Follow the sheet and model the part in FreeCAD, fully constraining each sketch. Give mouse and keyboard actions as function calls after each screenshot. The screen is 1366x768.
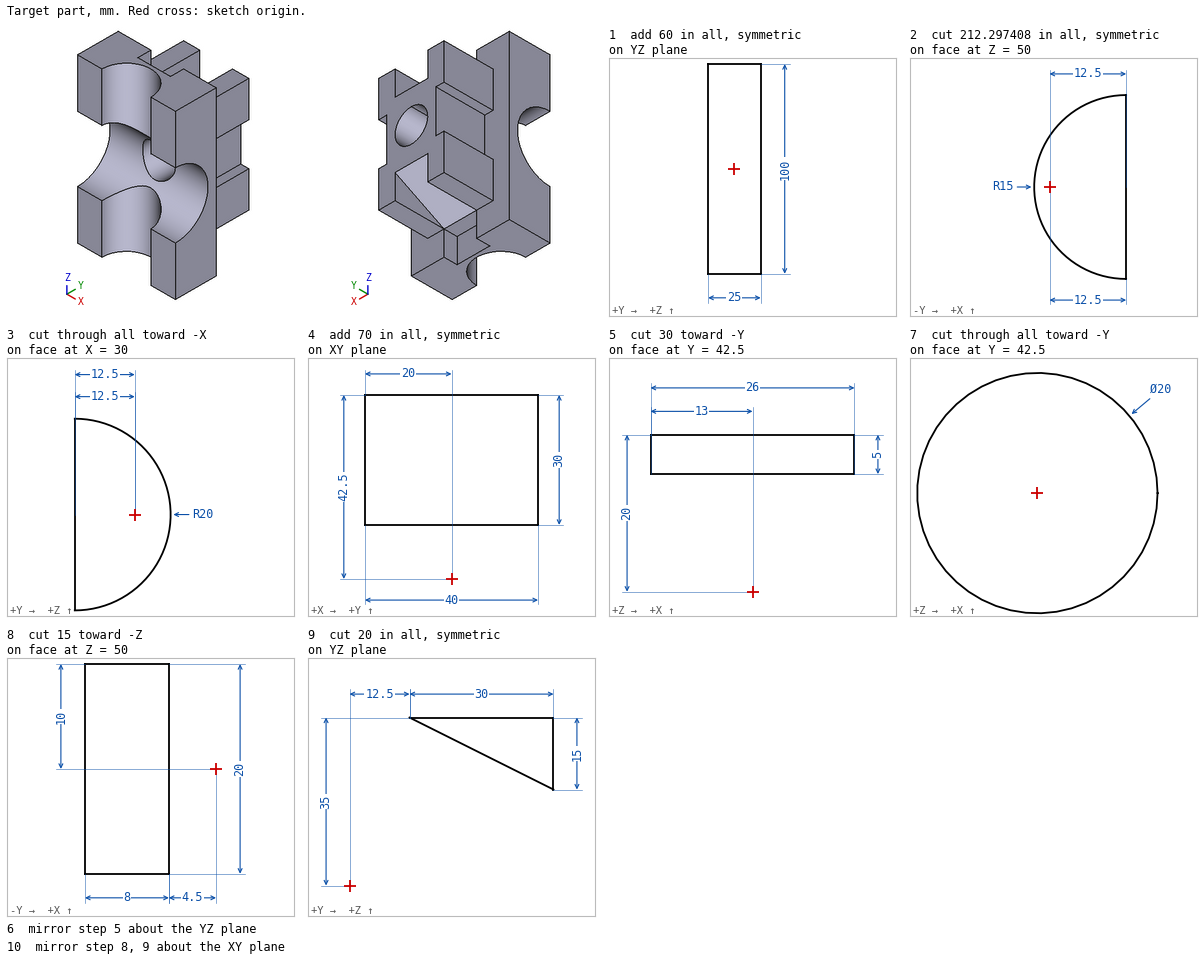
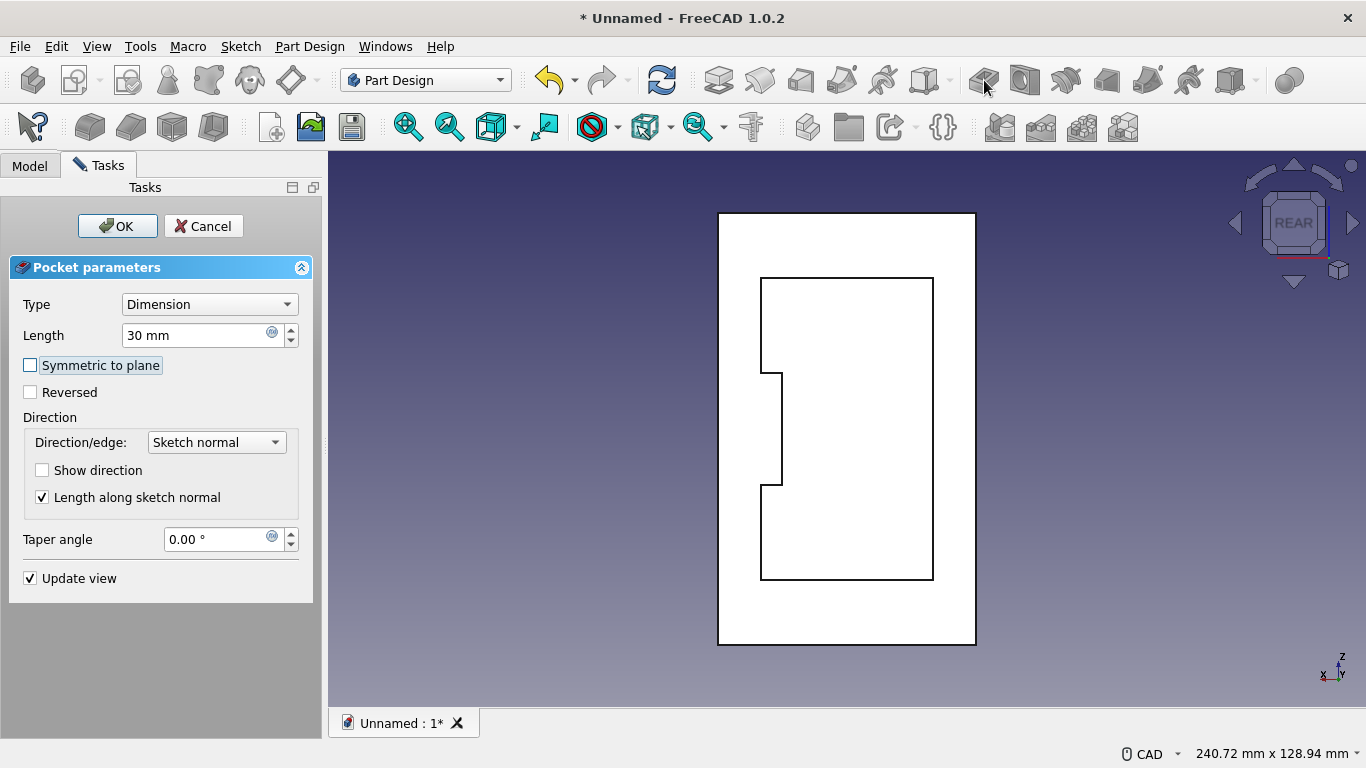
click(118, 226)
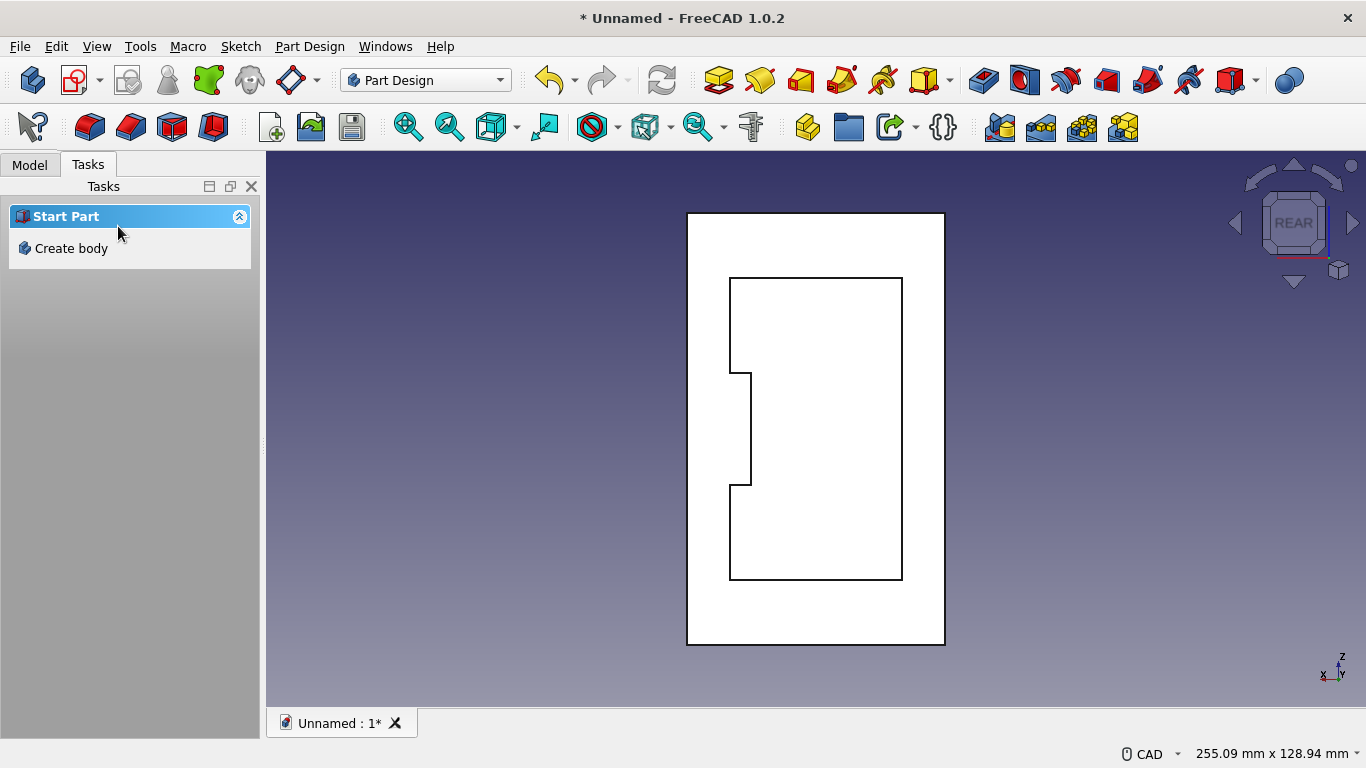
click(30, 164)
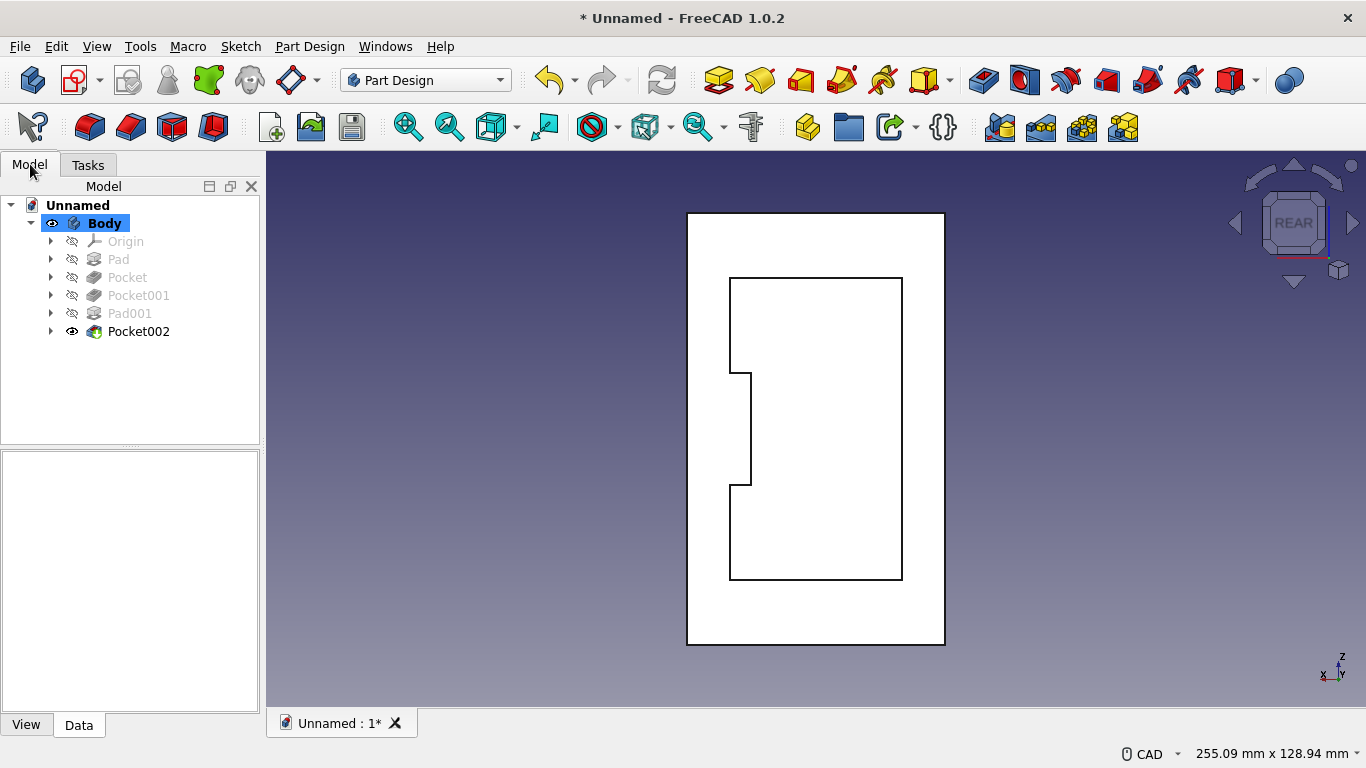
click(117, 331)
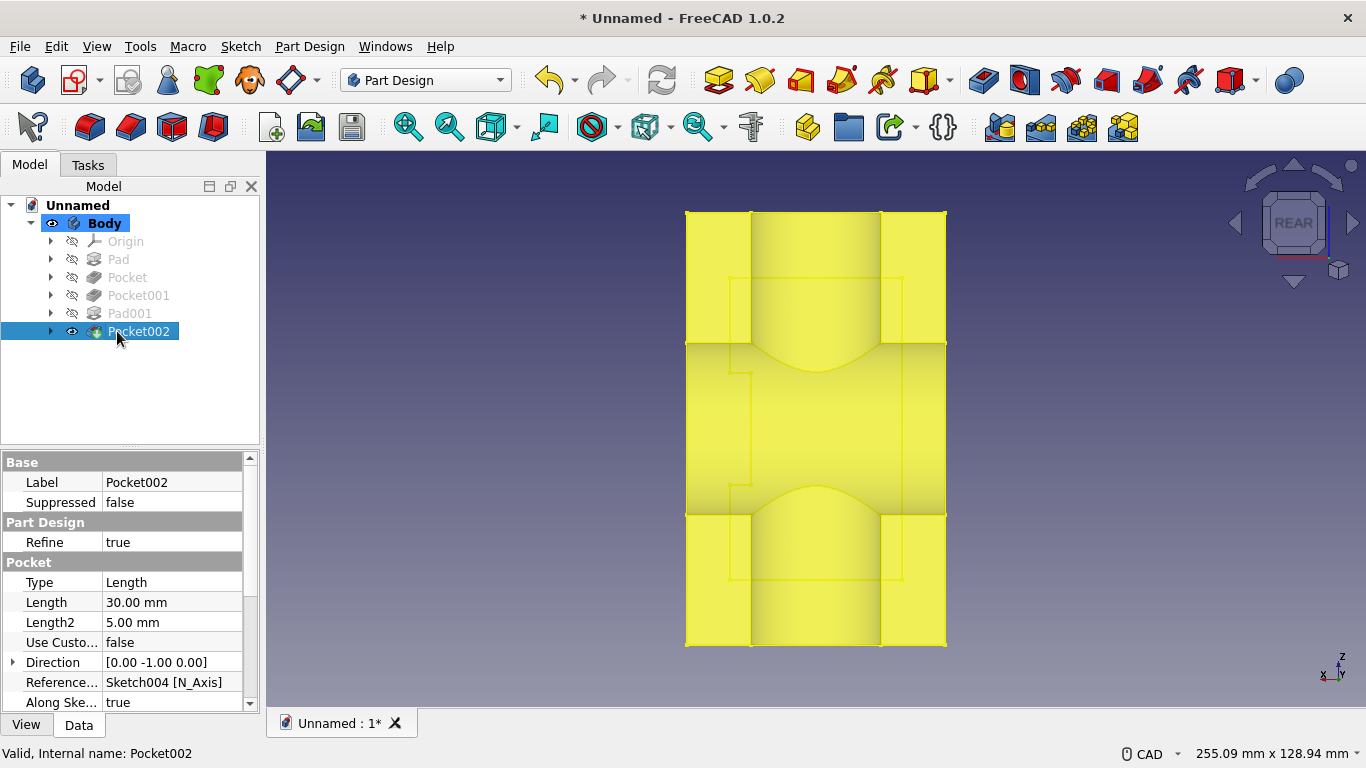
click(1000, 128)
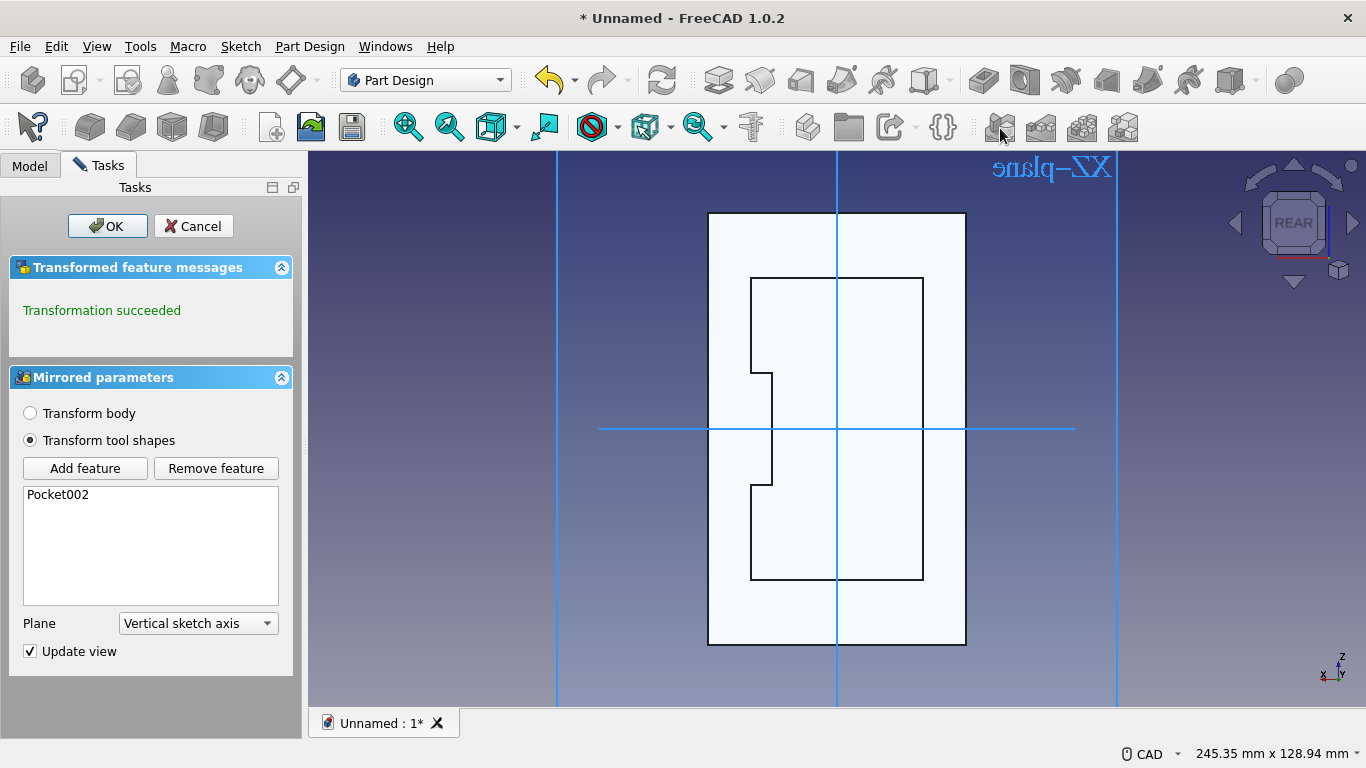
click(199, 624)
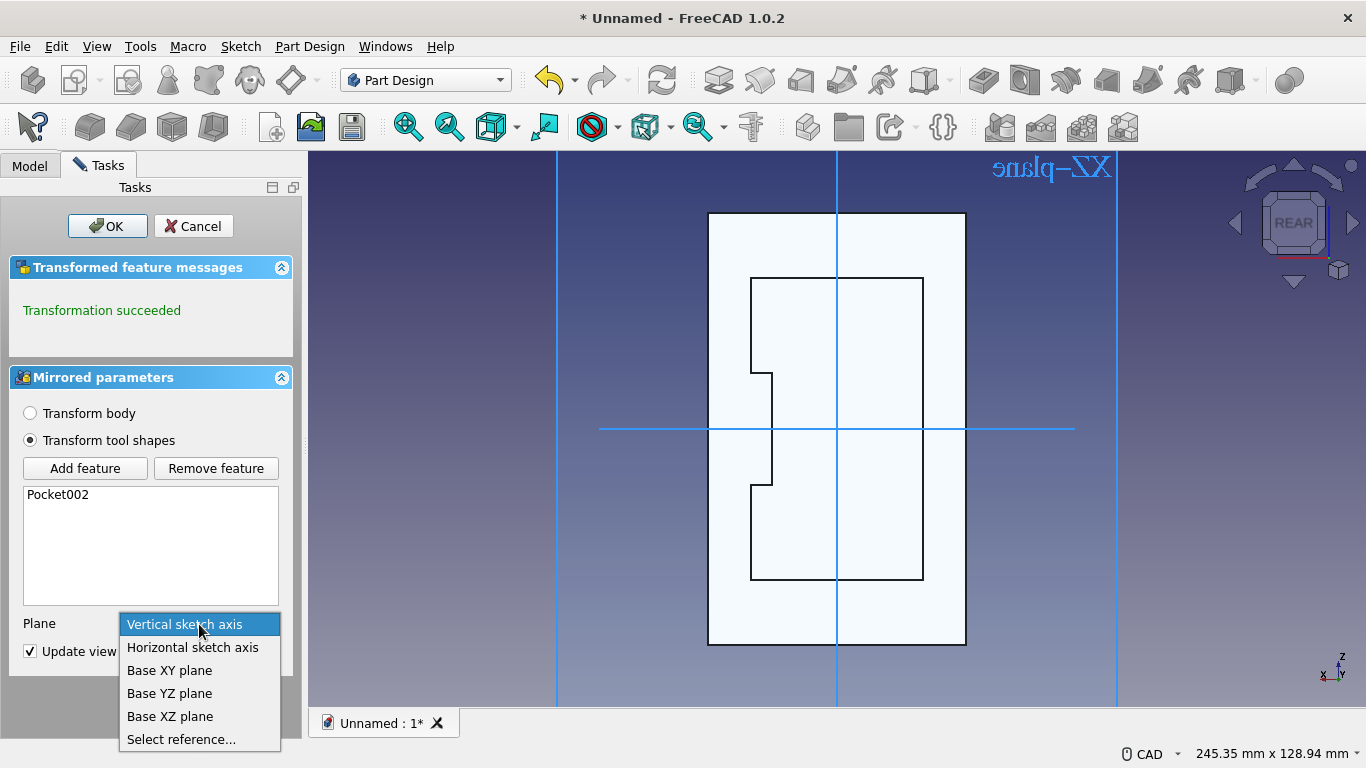
click(198, 694)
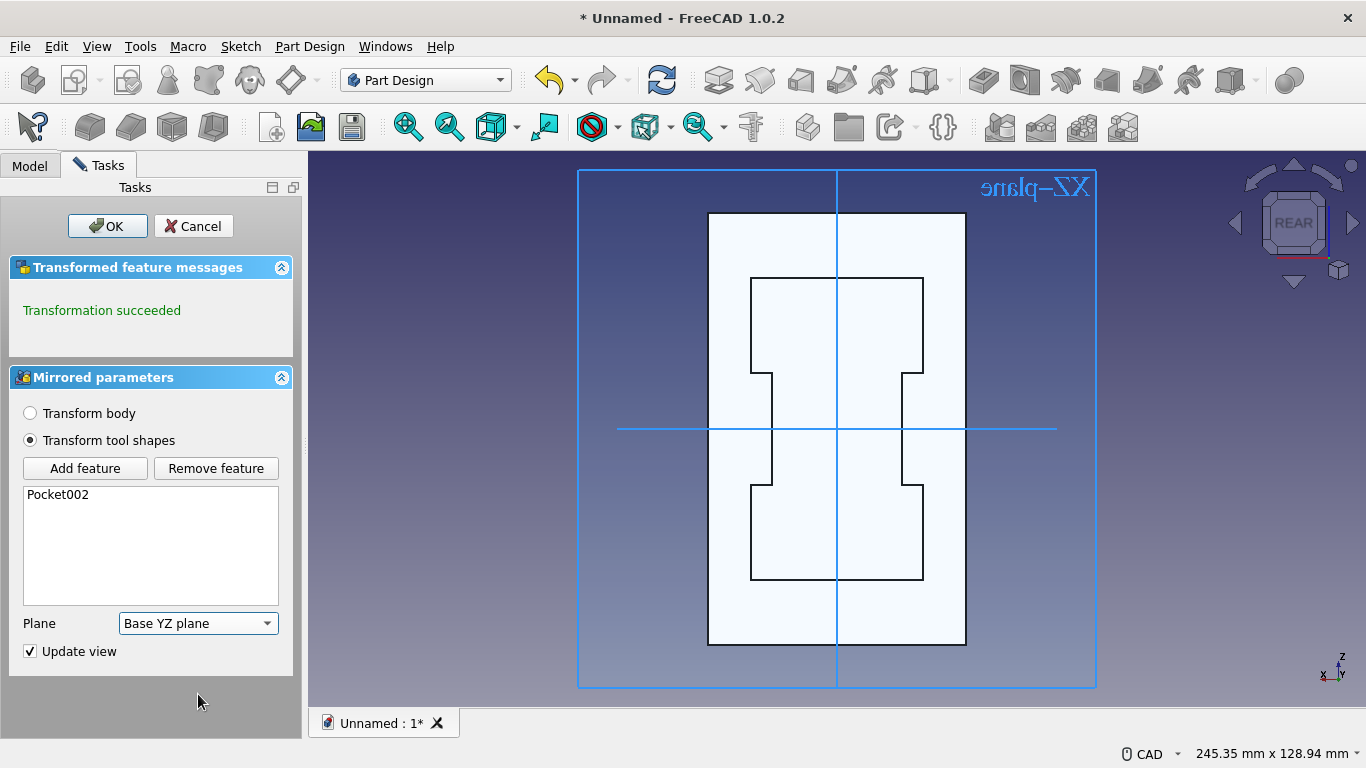
click(108, 226)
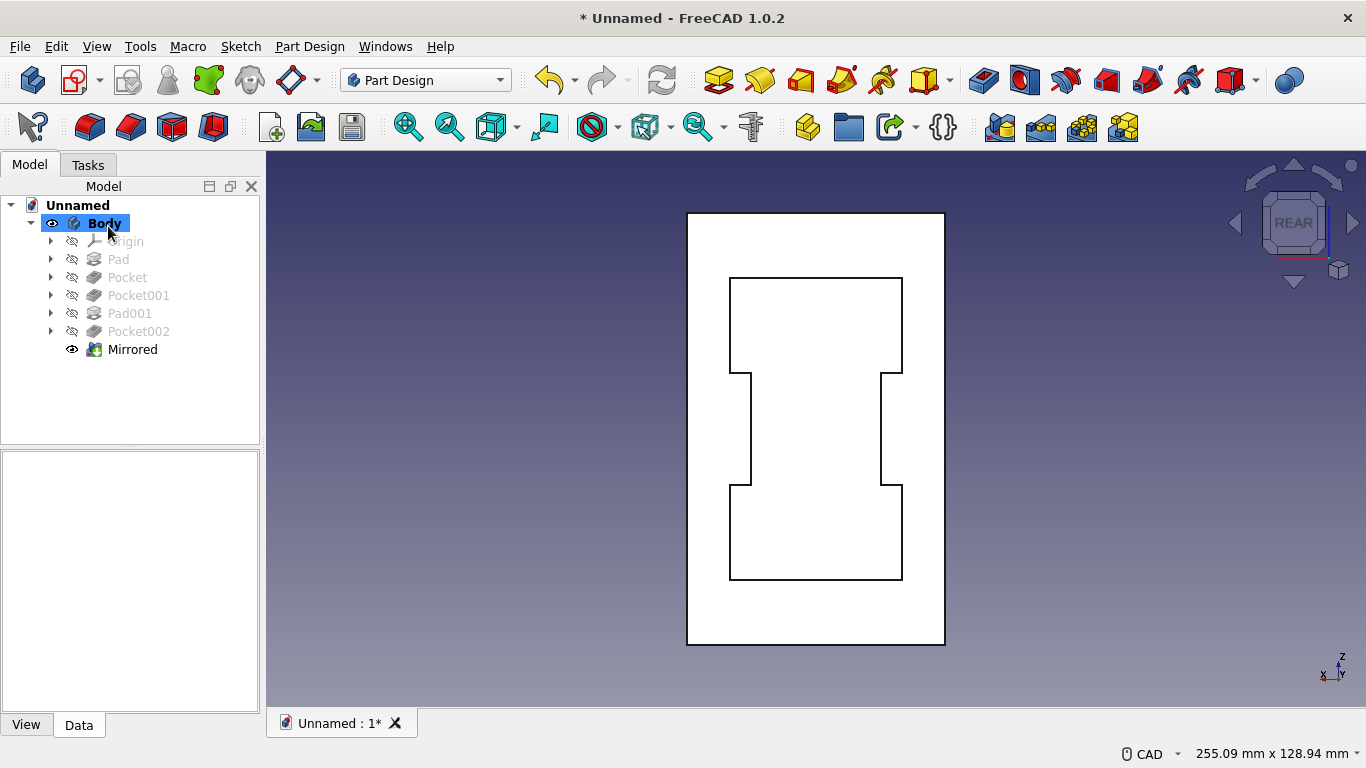
click(816, 514)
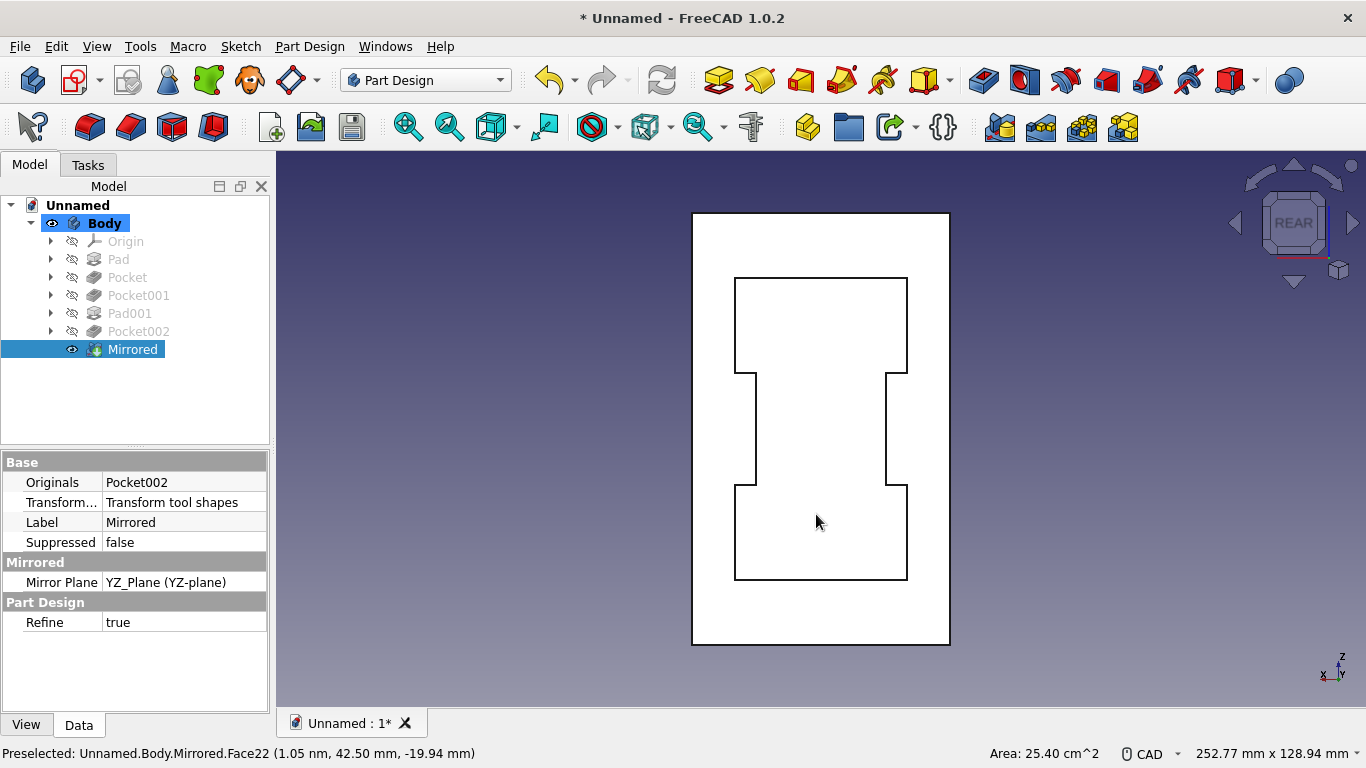
click(74, 80)